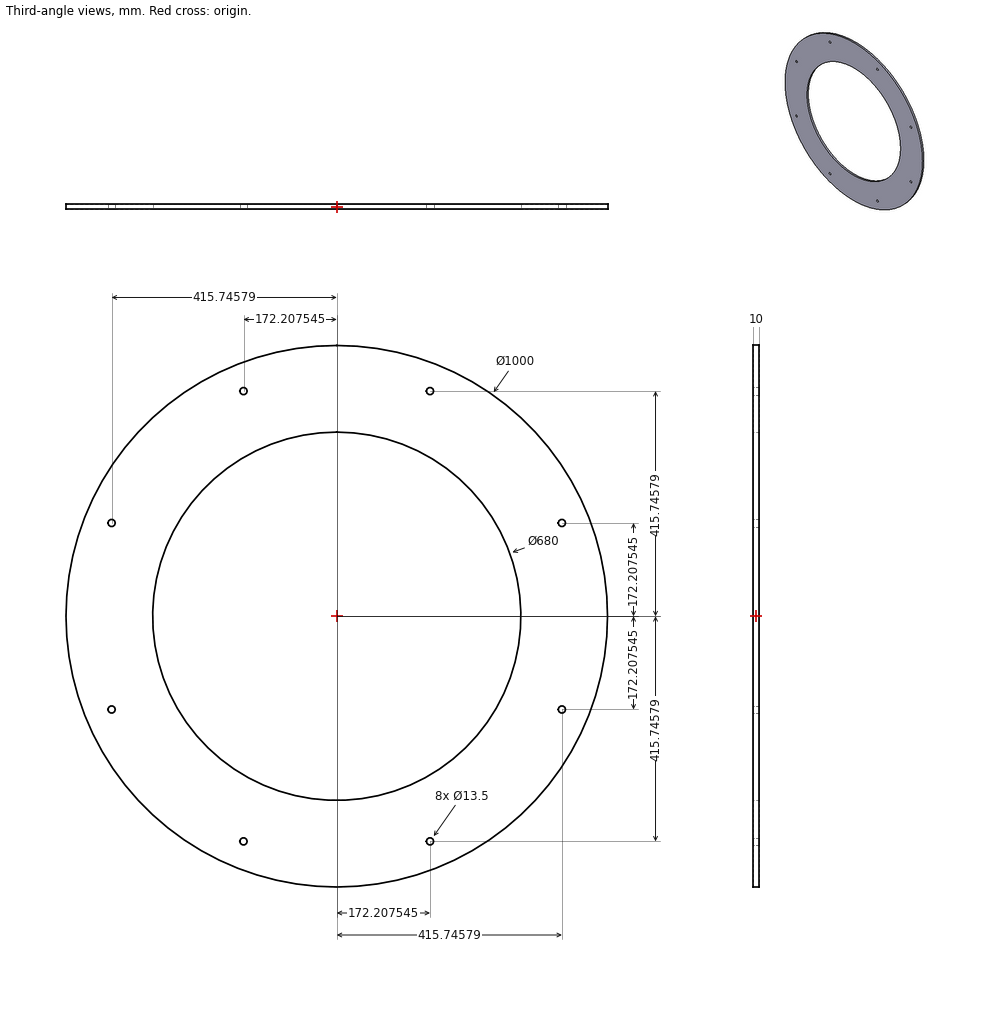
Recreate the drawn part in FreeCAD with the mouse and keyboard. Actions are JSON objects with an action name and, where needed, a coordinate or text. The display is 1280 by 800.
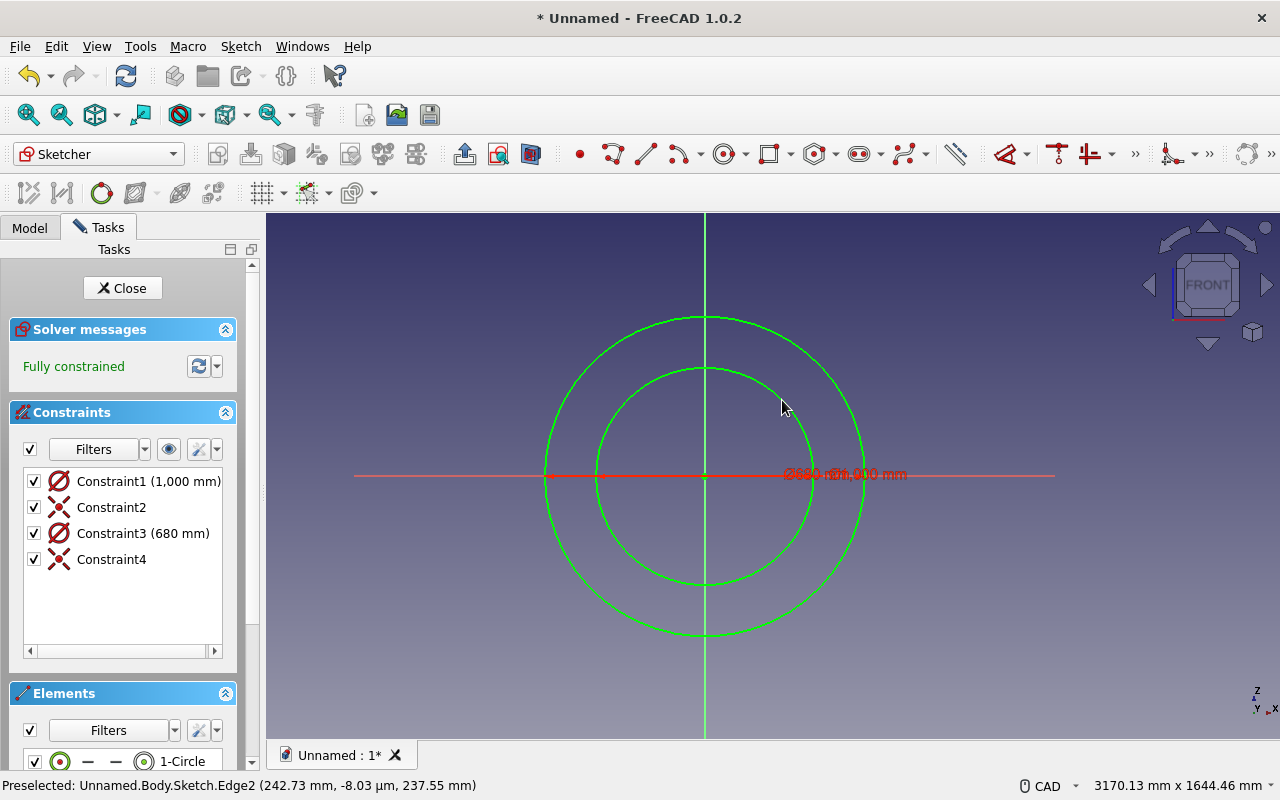
{"action": "left_click", "coordinate": [123, 288]}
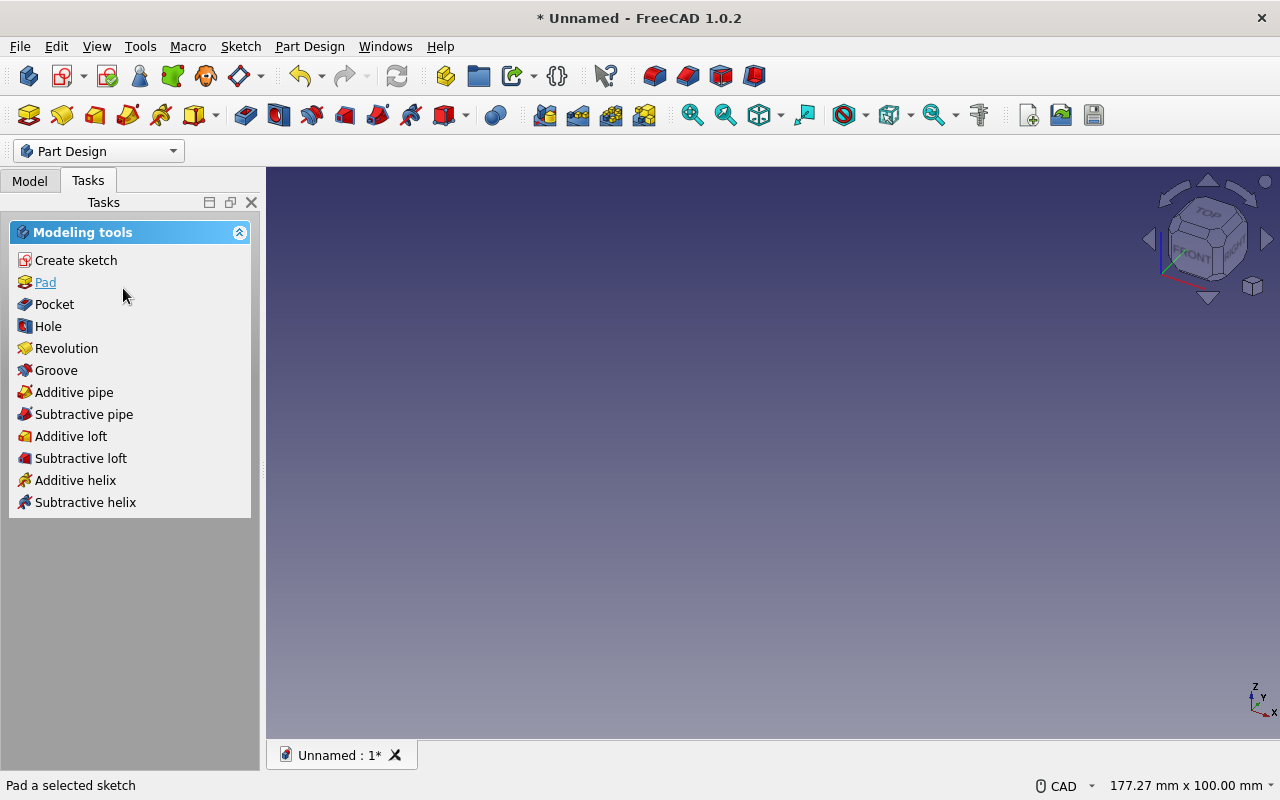
{"action": "left_click", "coordinate": [29, 116]}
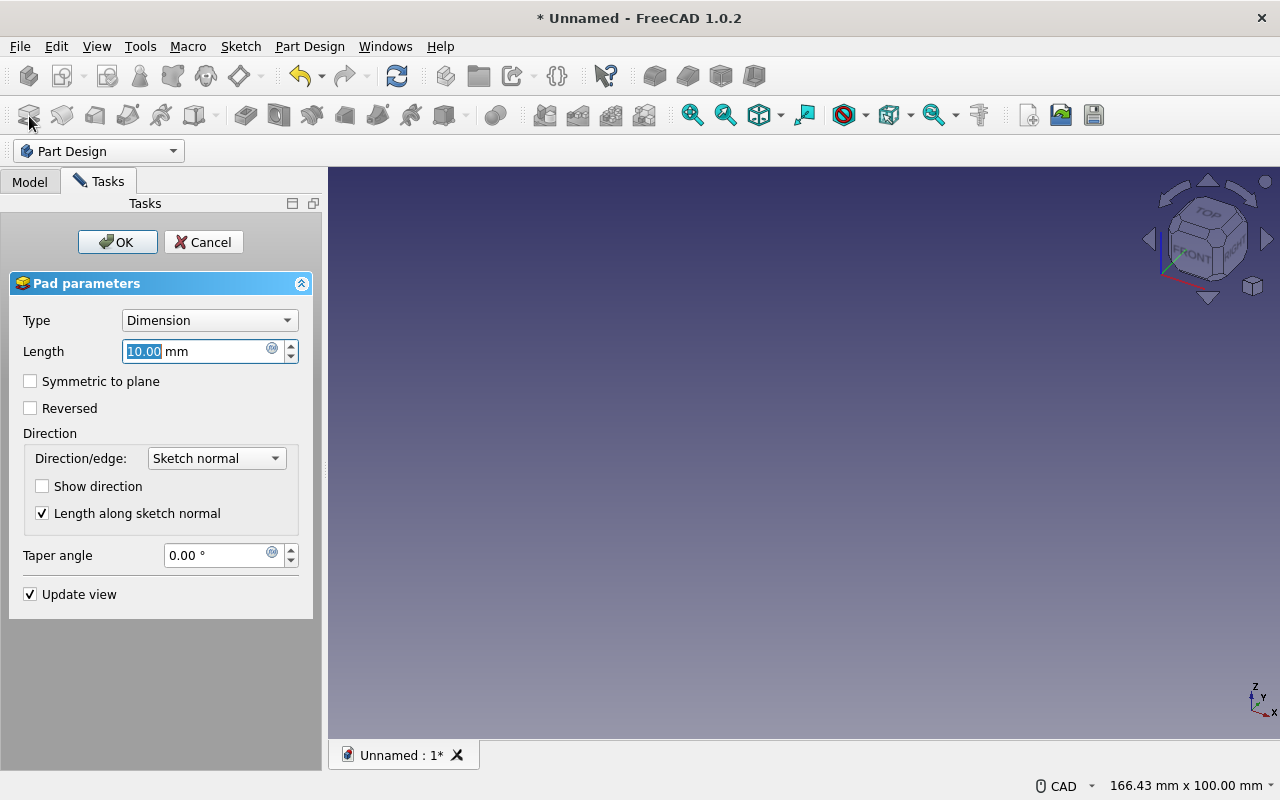
{"action": "type", "text": "10"}
{"action": "key", "text": "Tab"}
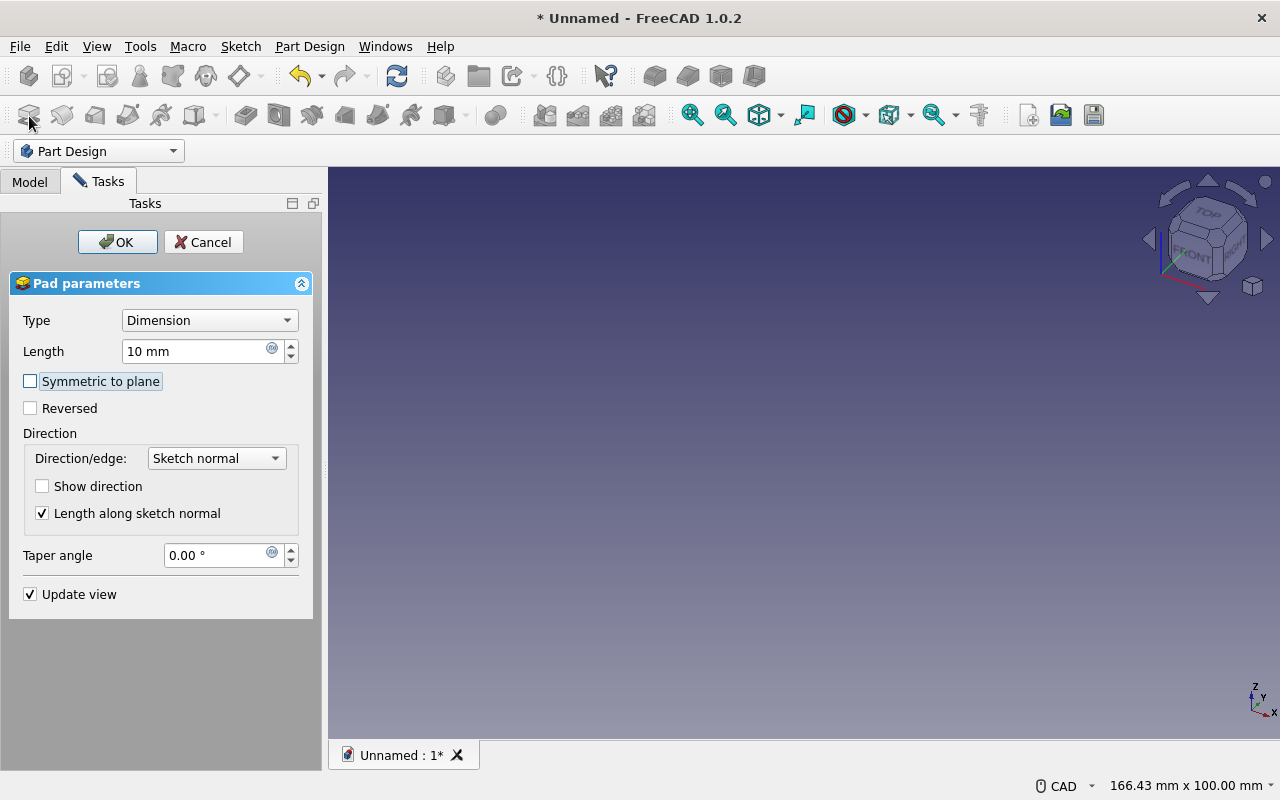
{"action": "left_click", "coordinate": [31, 381]}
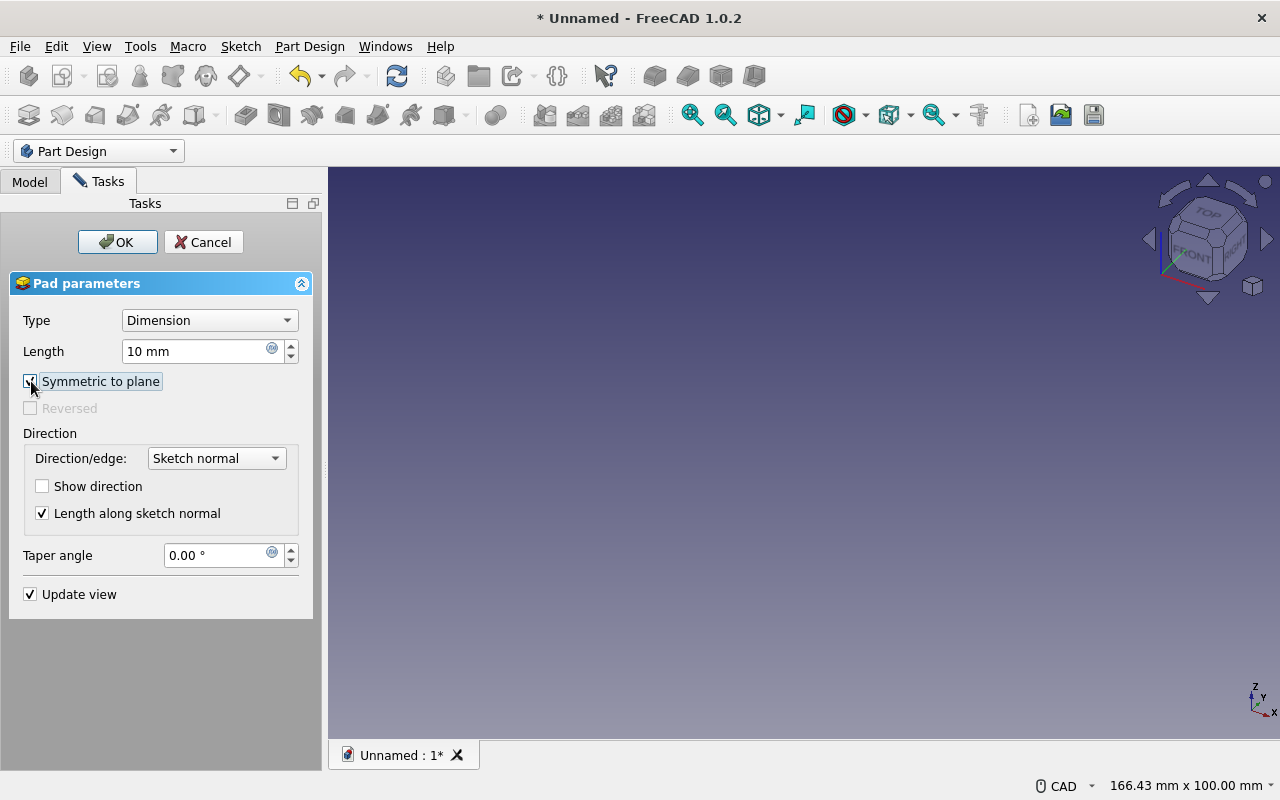
{"action": "left_click", "coordinate": [118, 242]}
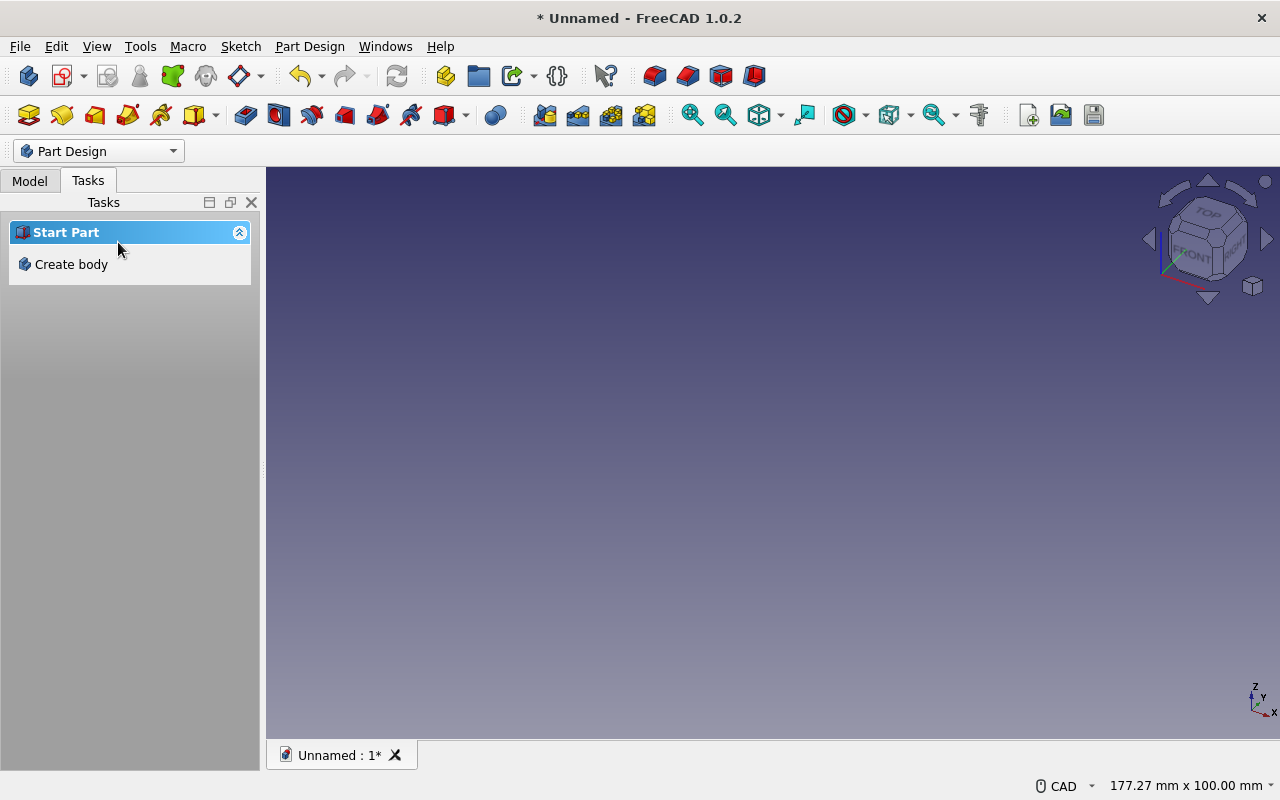
{"action": "key", "text": "v f"}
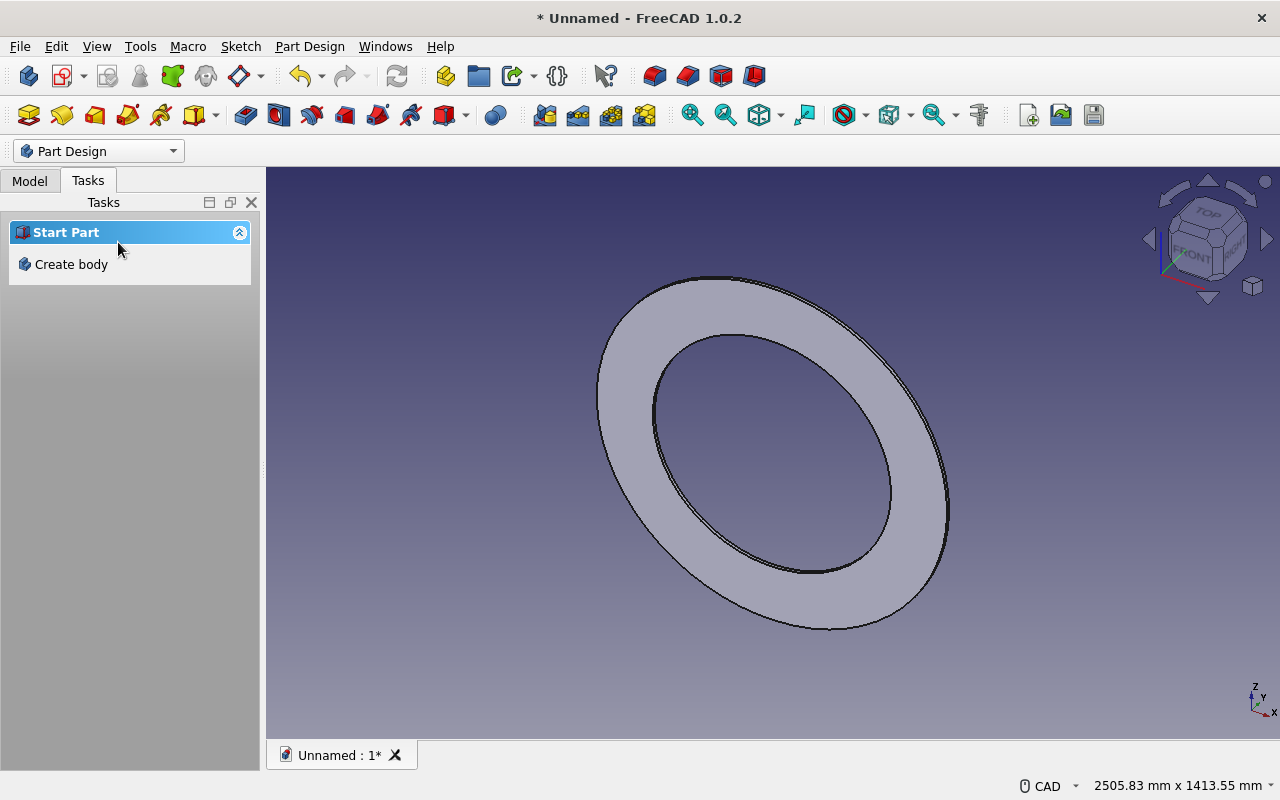
{"action": "key", "text": "4"}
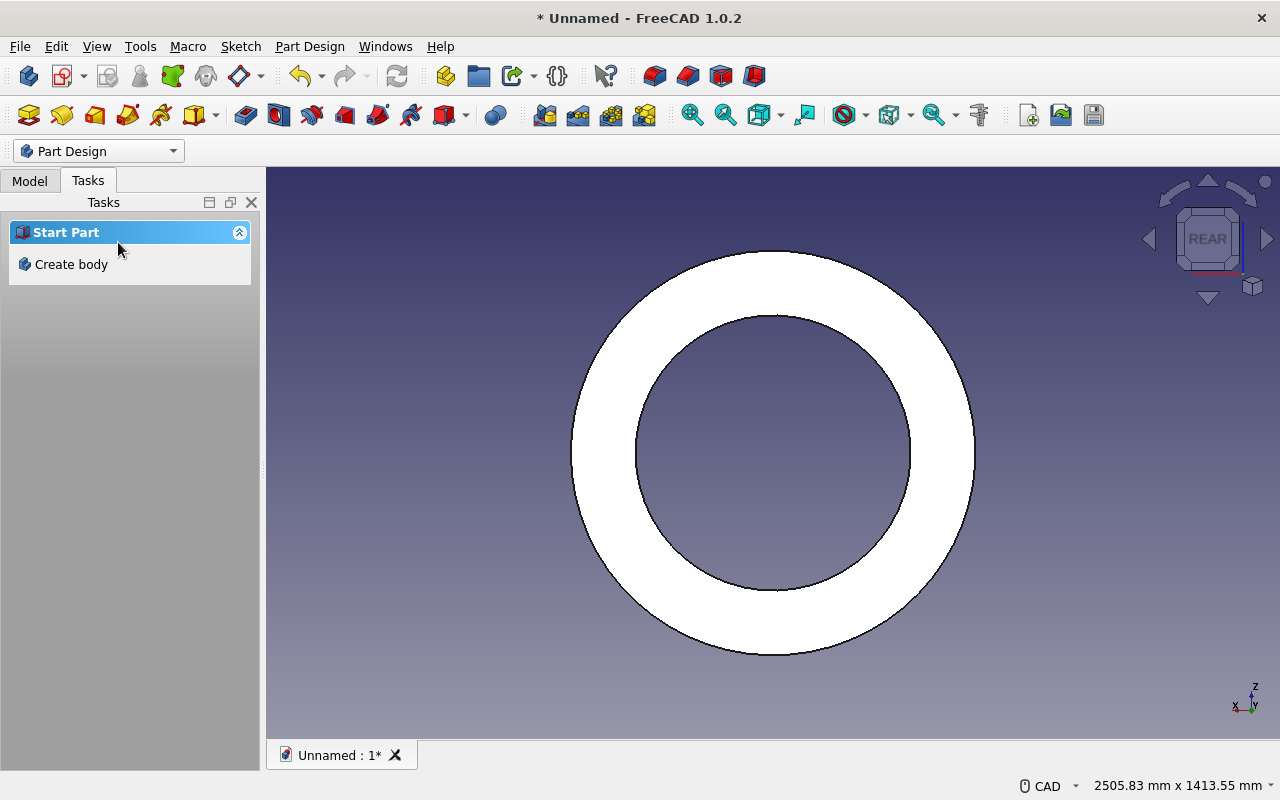
{"action": "left_click", "coordinate": [600, 452]}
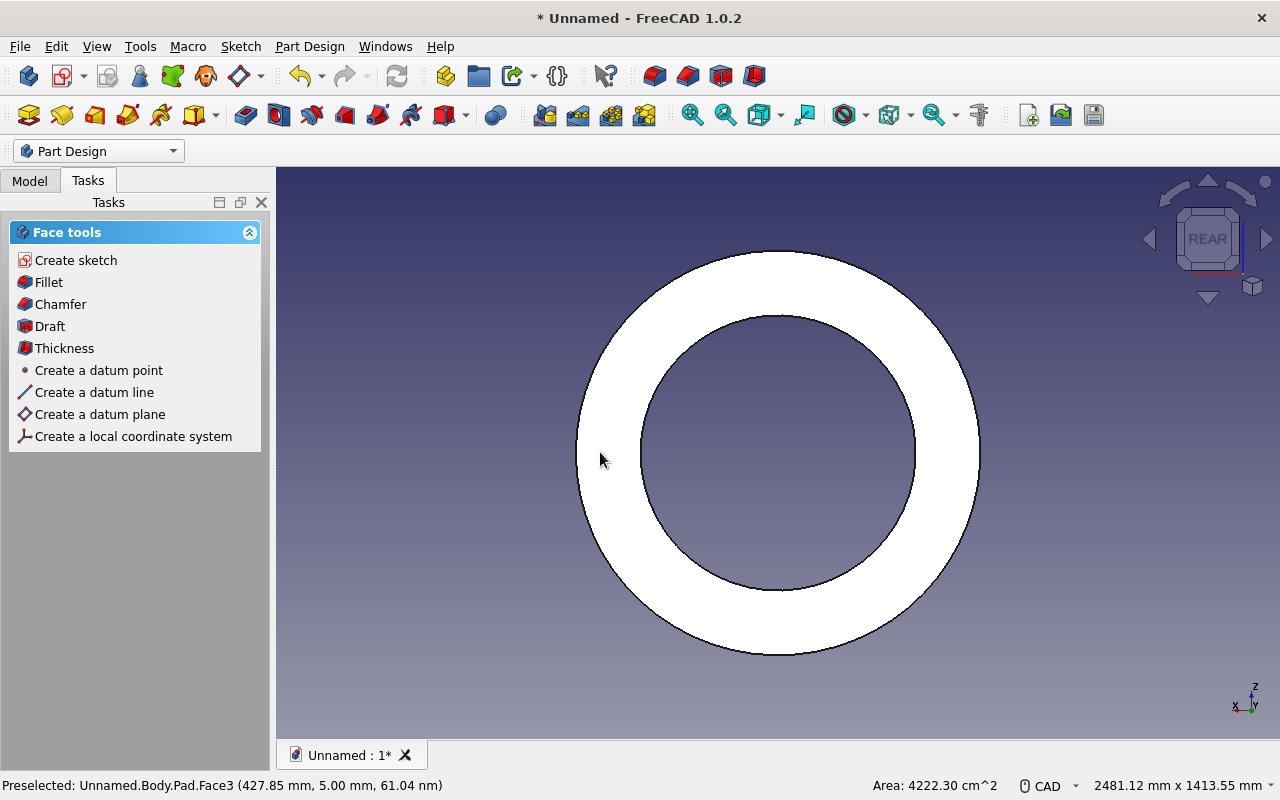
{"action": "left_click", "coordinate": [62, 76]}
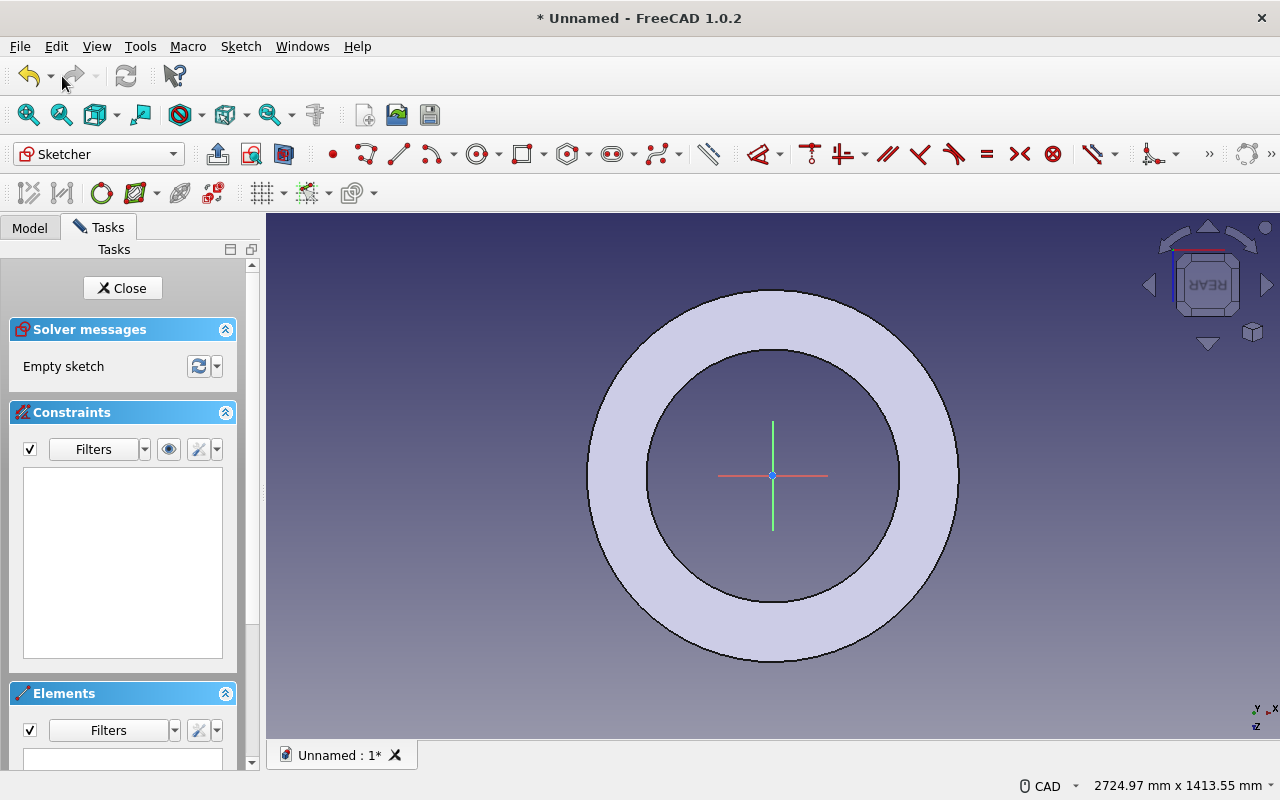
{"action": "left_click", "coordinate": [476, 154]}